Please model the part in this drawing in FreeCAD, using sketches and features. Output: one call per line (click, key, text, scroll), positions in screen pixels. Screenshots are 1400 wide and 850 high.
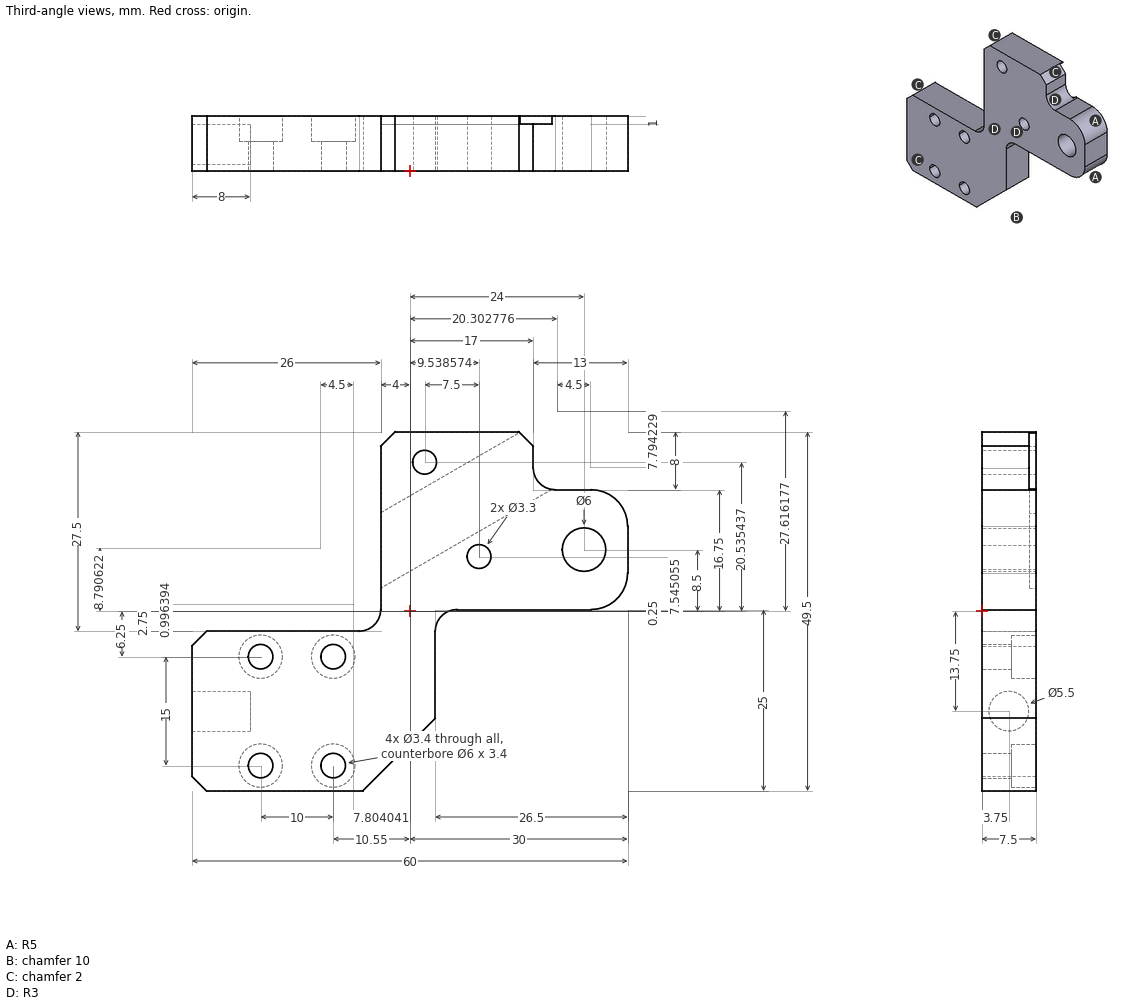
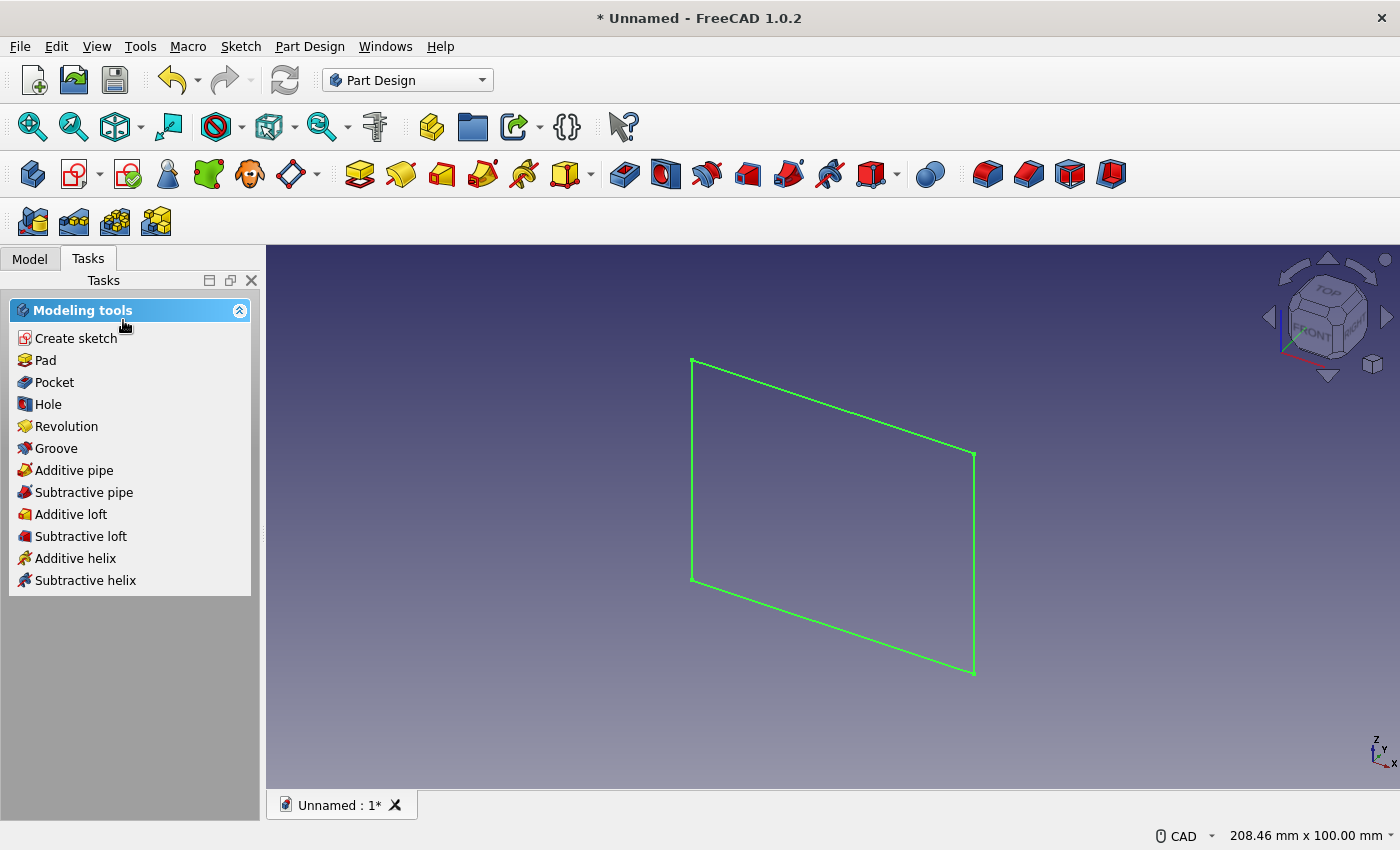
click(360, 174)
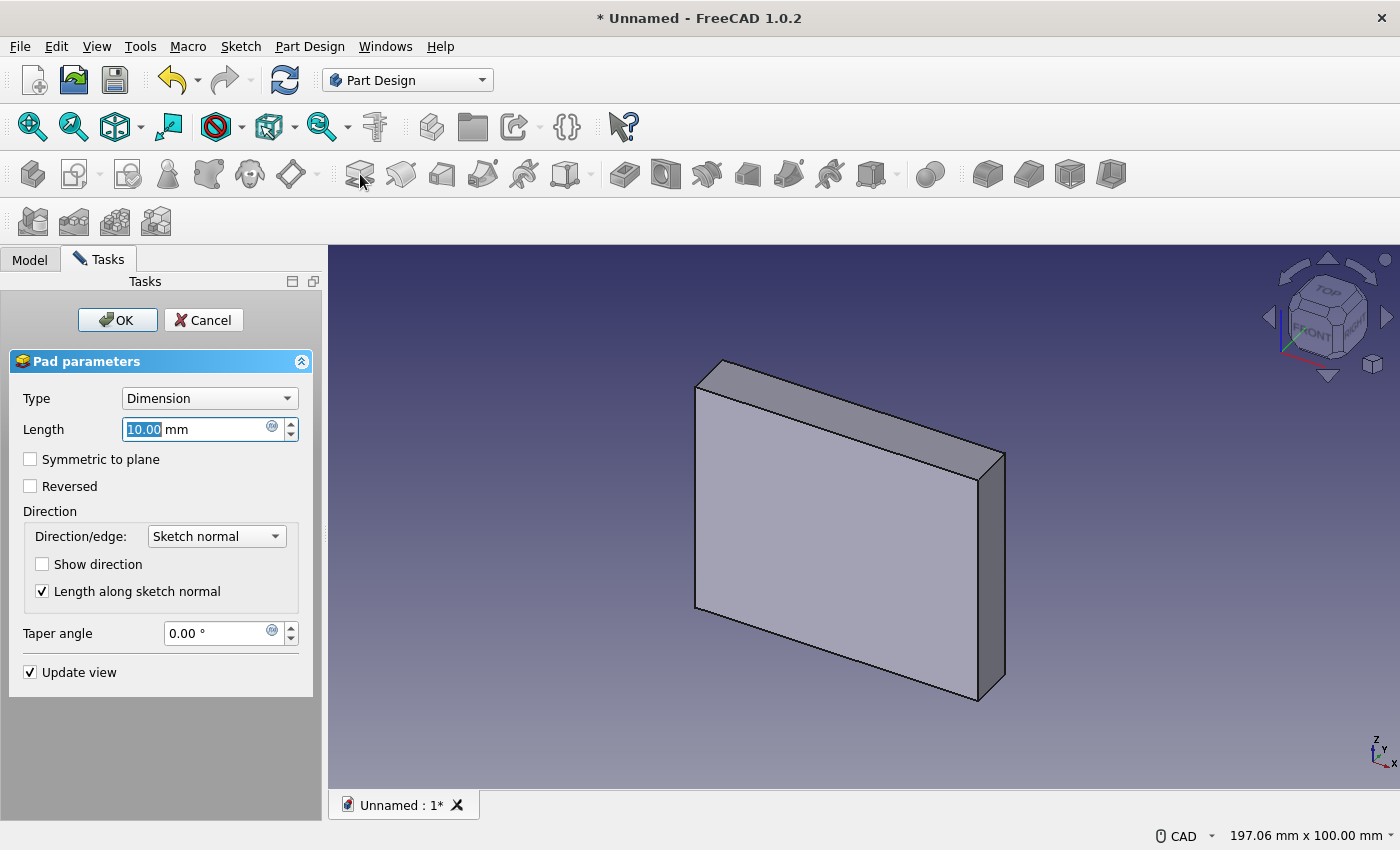
text(7.5)
key(Tab)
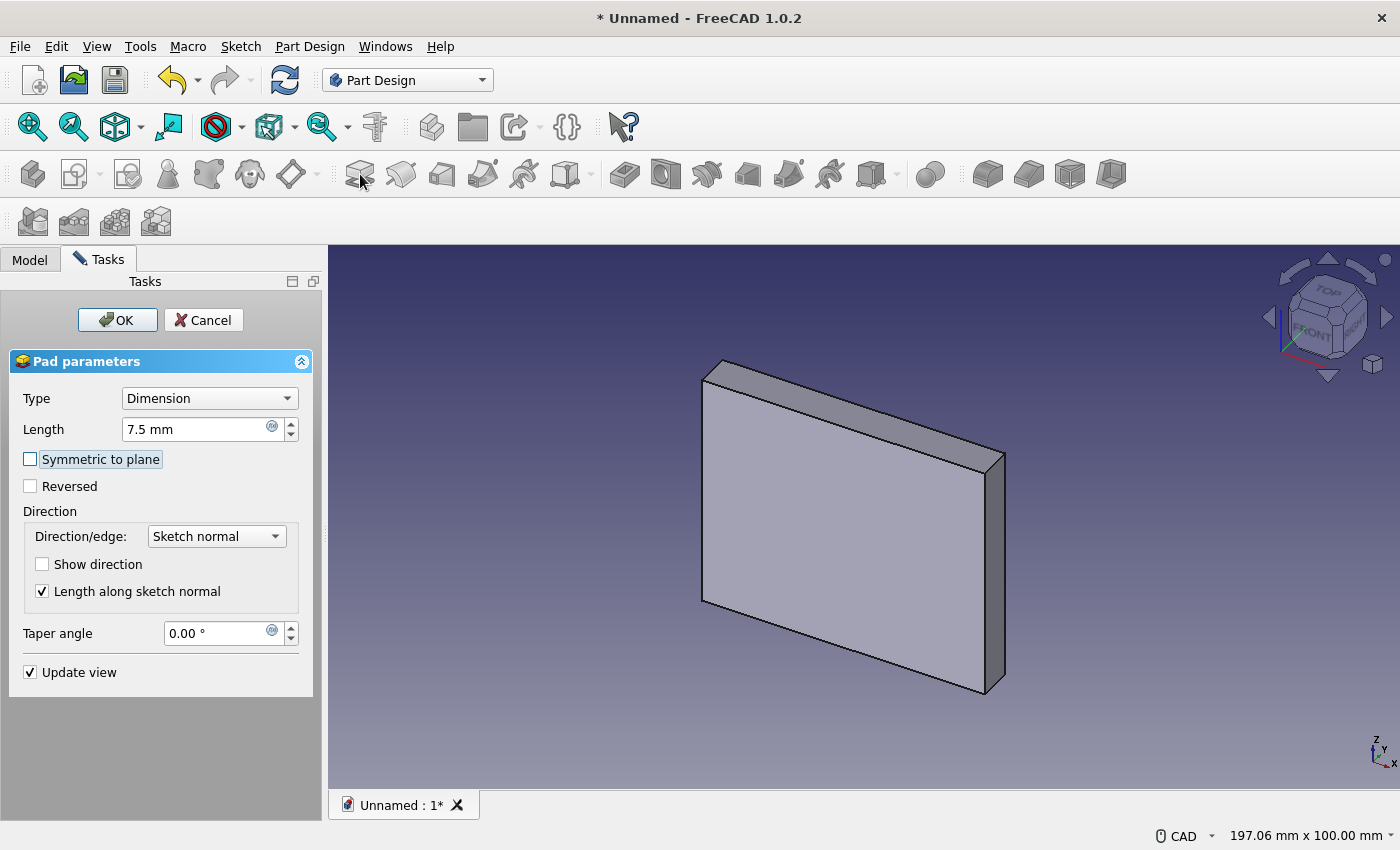
click(31, 486)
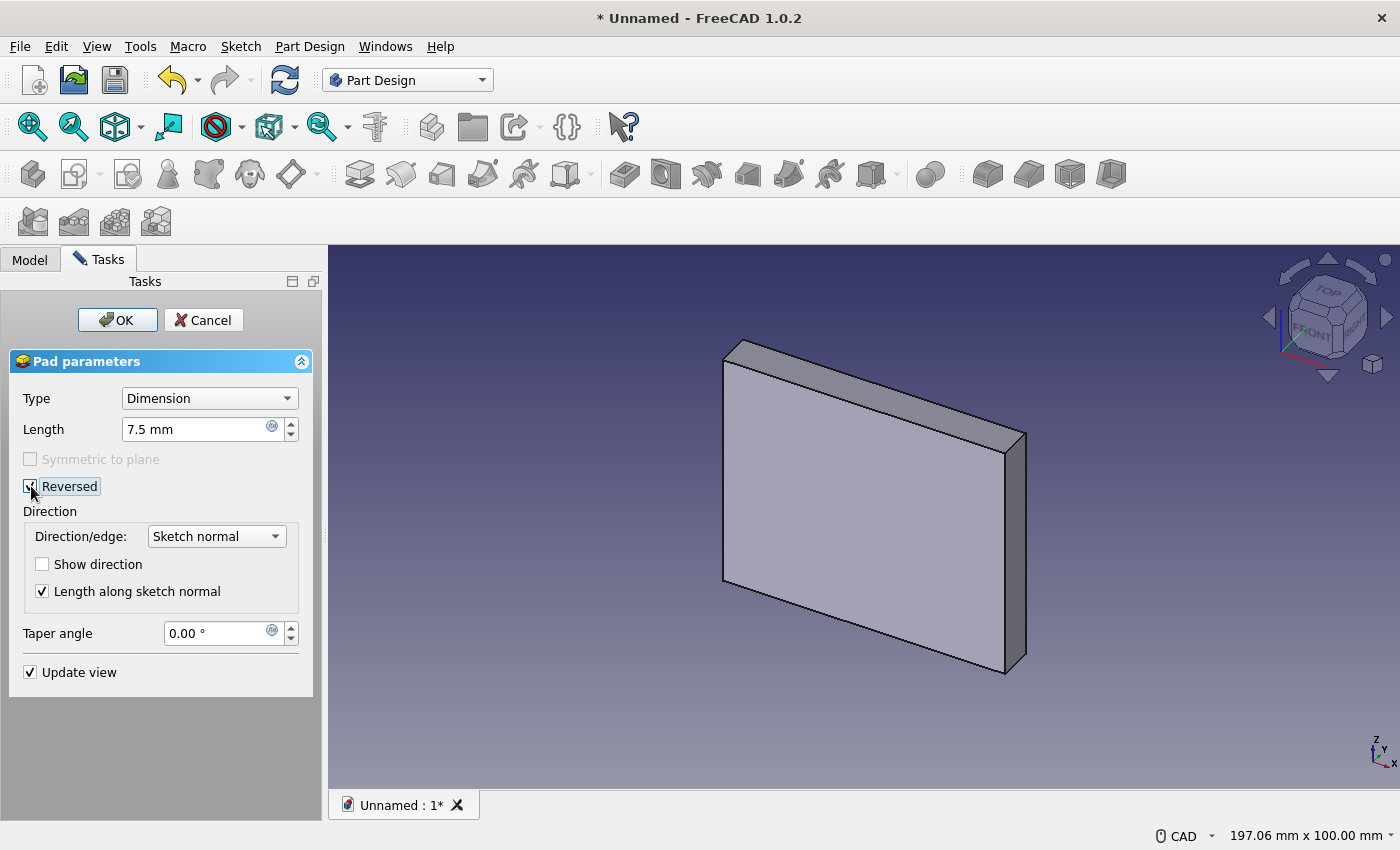
click(118, 320)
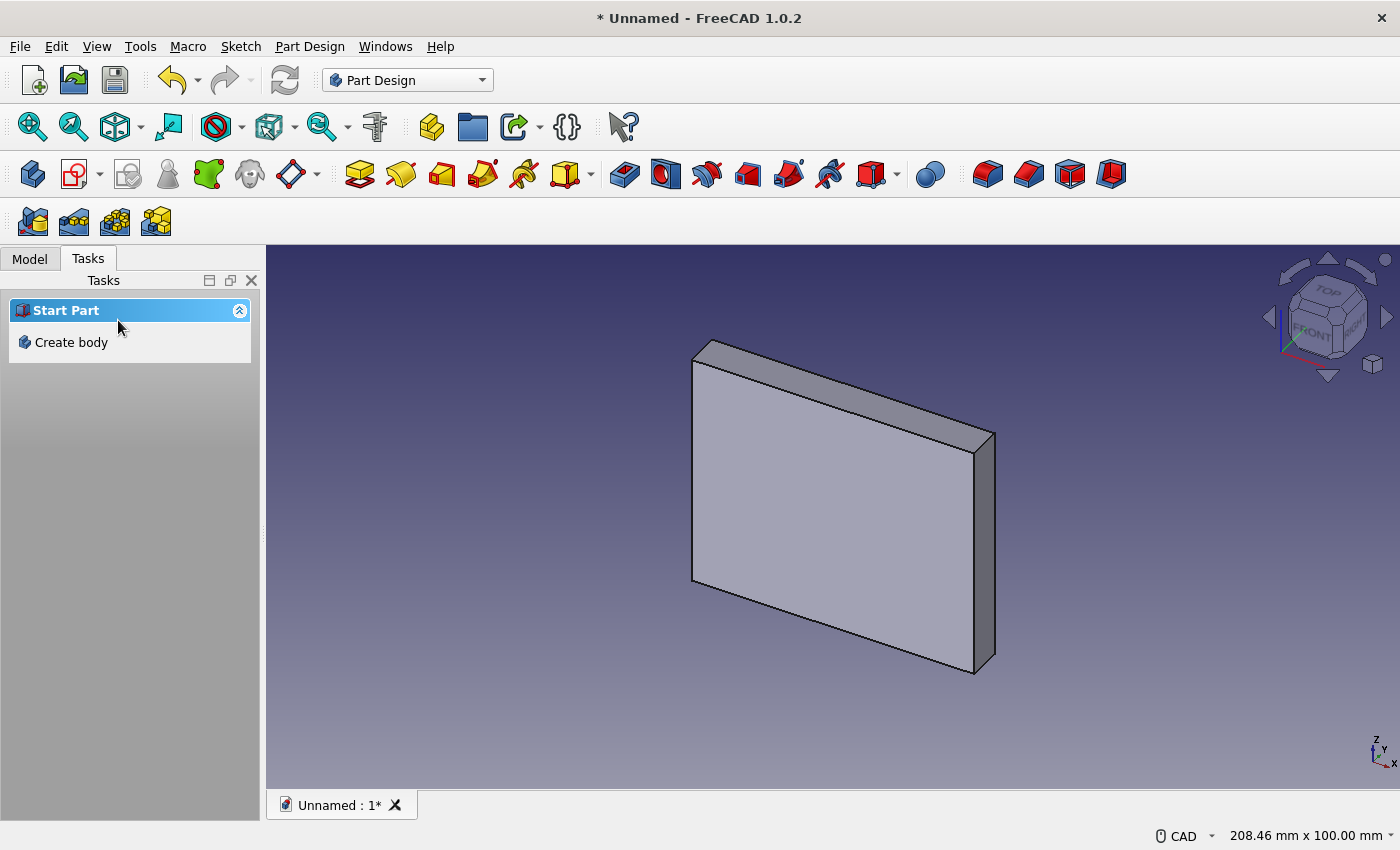
key(4)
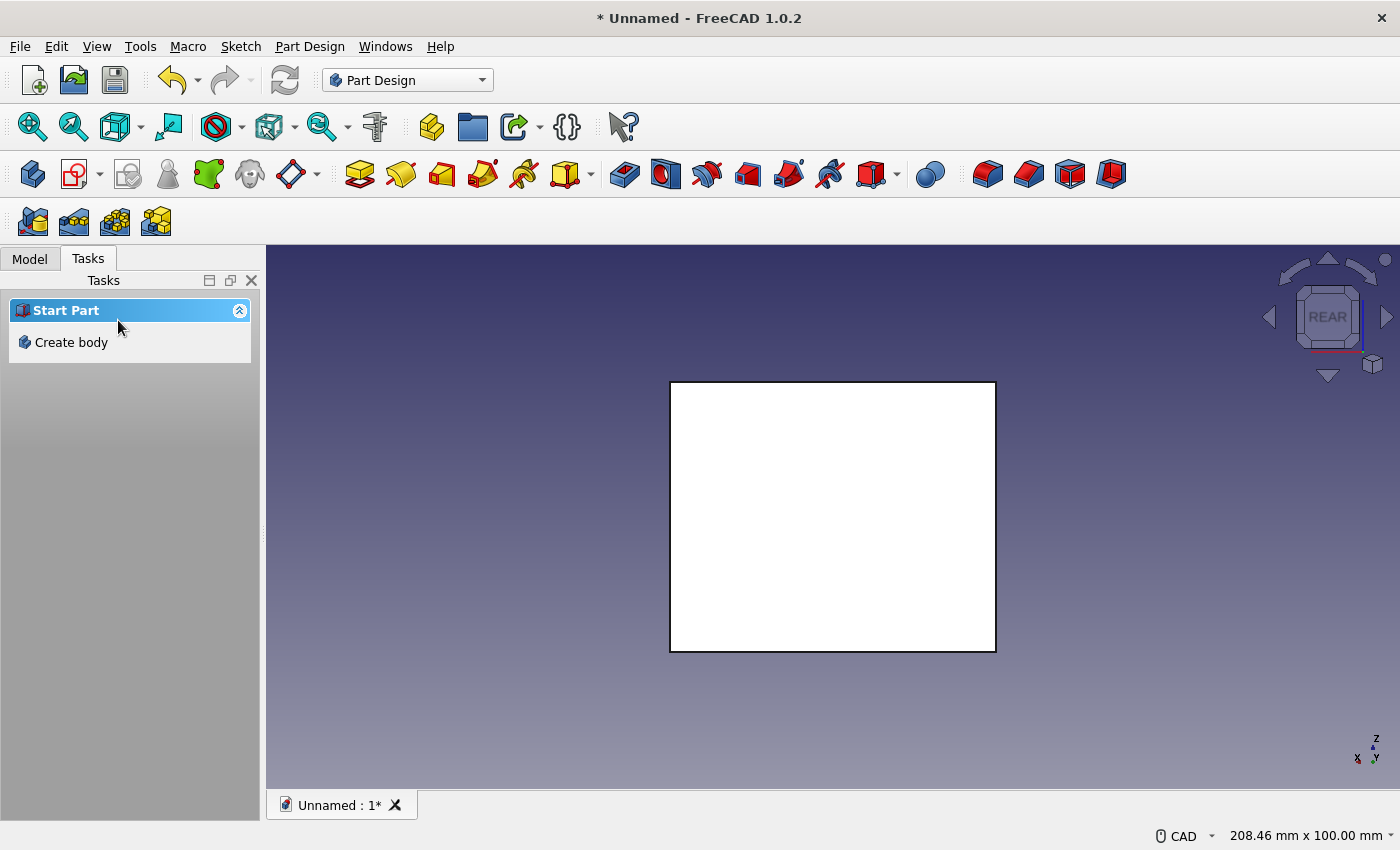
click(833, 516)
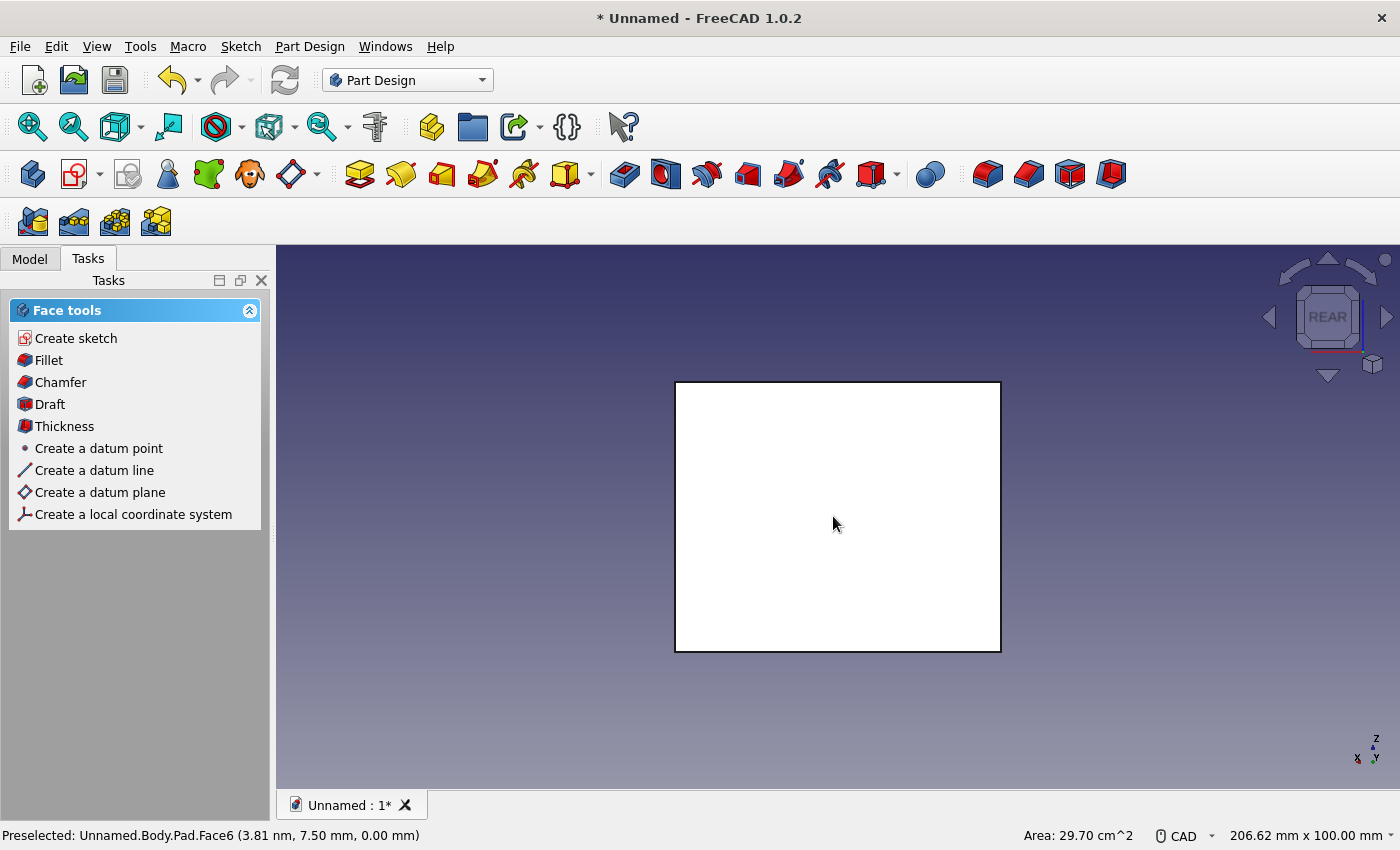
click(74, 174)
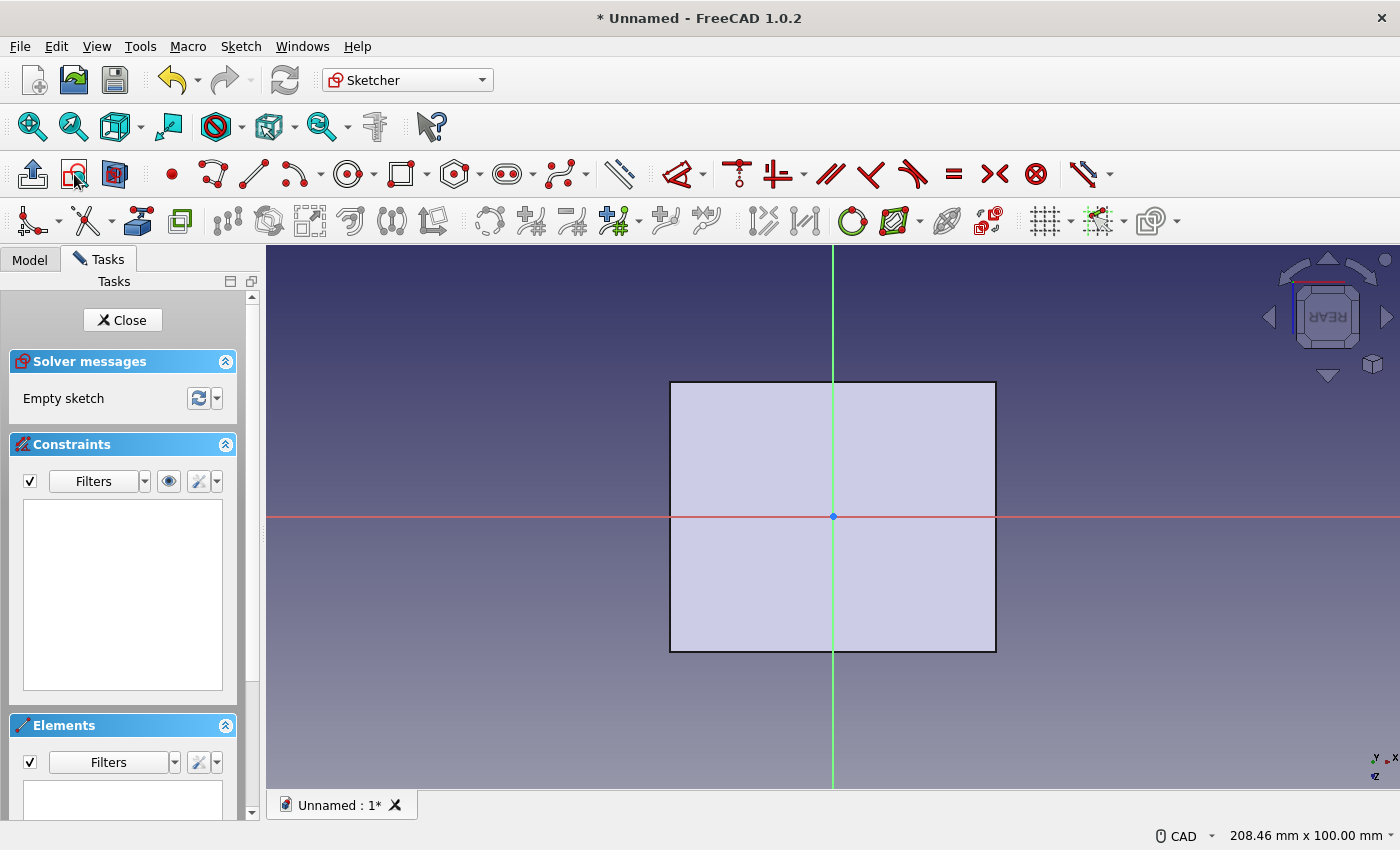
key(g)
key(r)